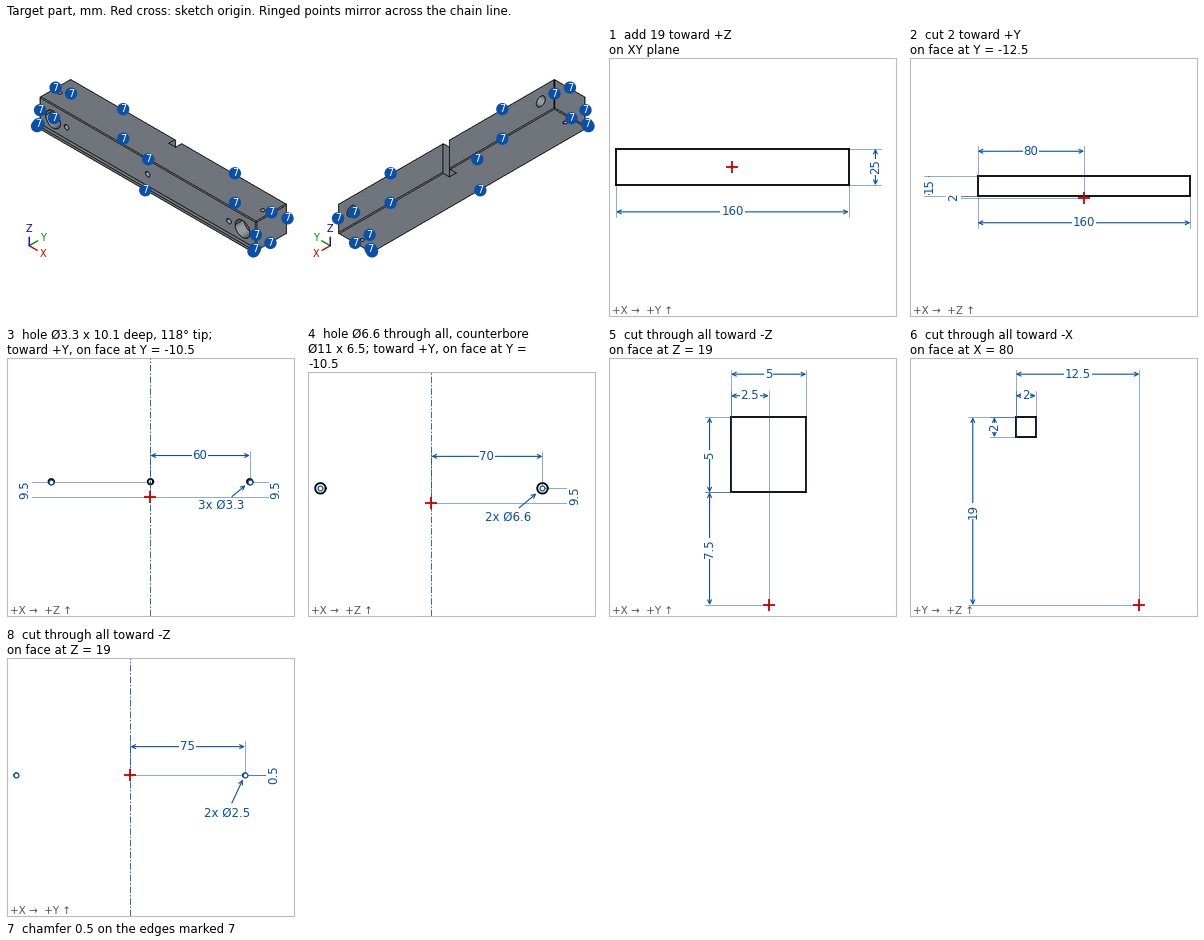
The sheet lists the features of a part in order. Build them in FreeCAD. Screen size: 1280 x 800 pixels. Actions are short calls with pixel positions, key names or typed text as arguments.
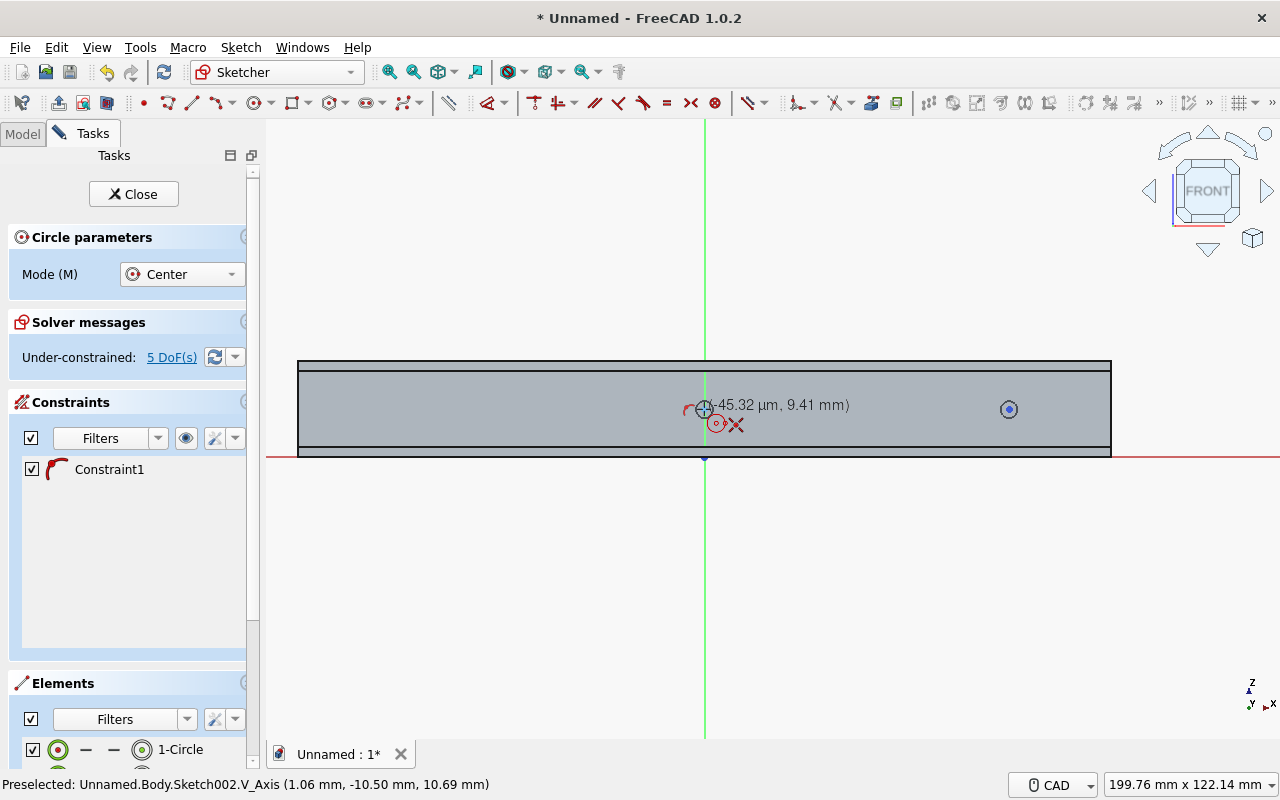
scroll(400, 409, up, 5)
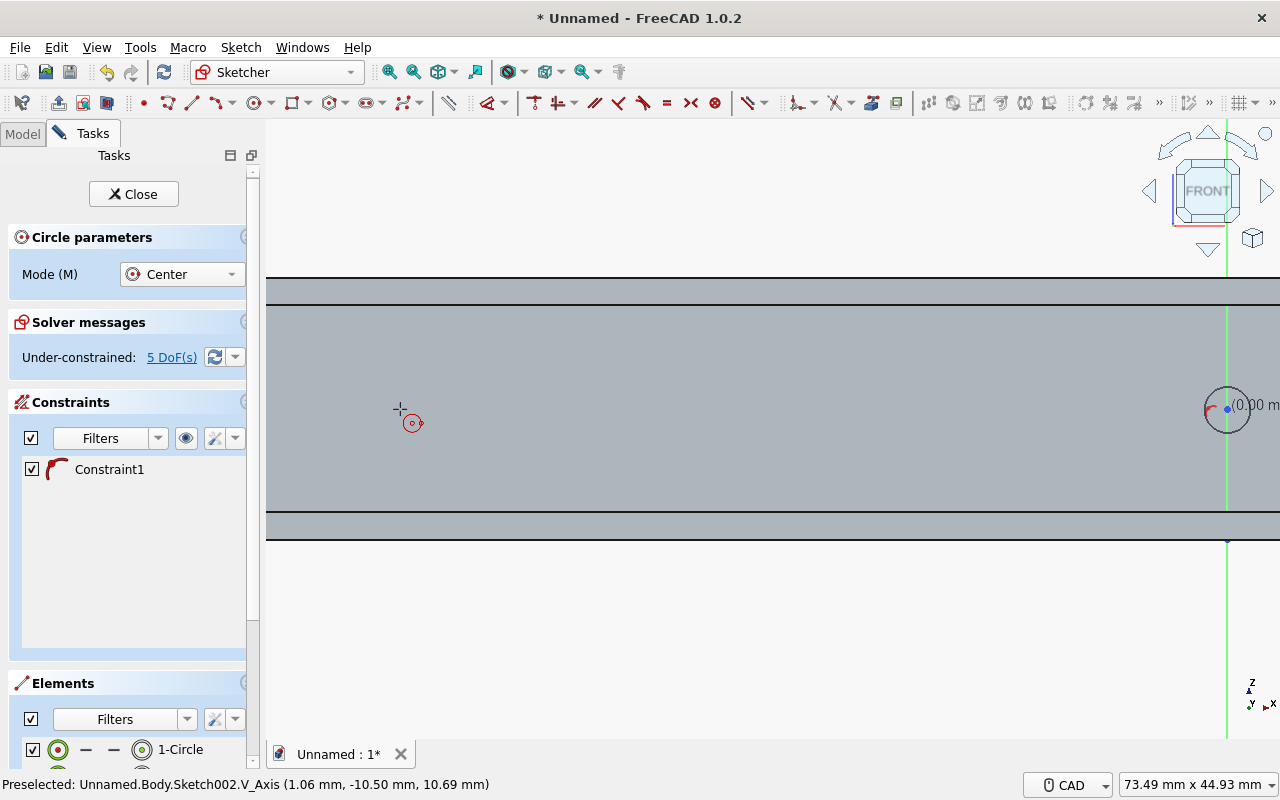
click(400, 409)
click(416, 393)
key(Escape)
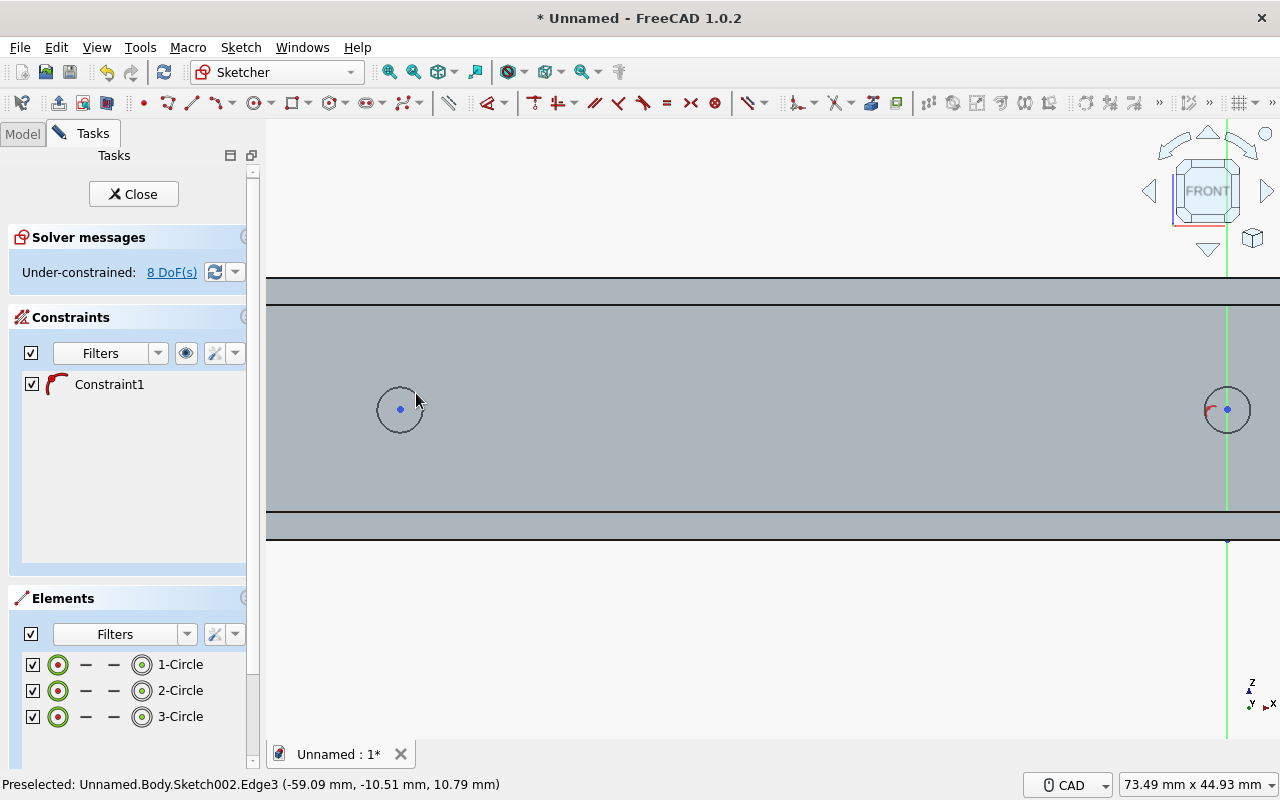
scroll(400, 409, down, 5)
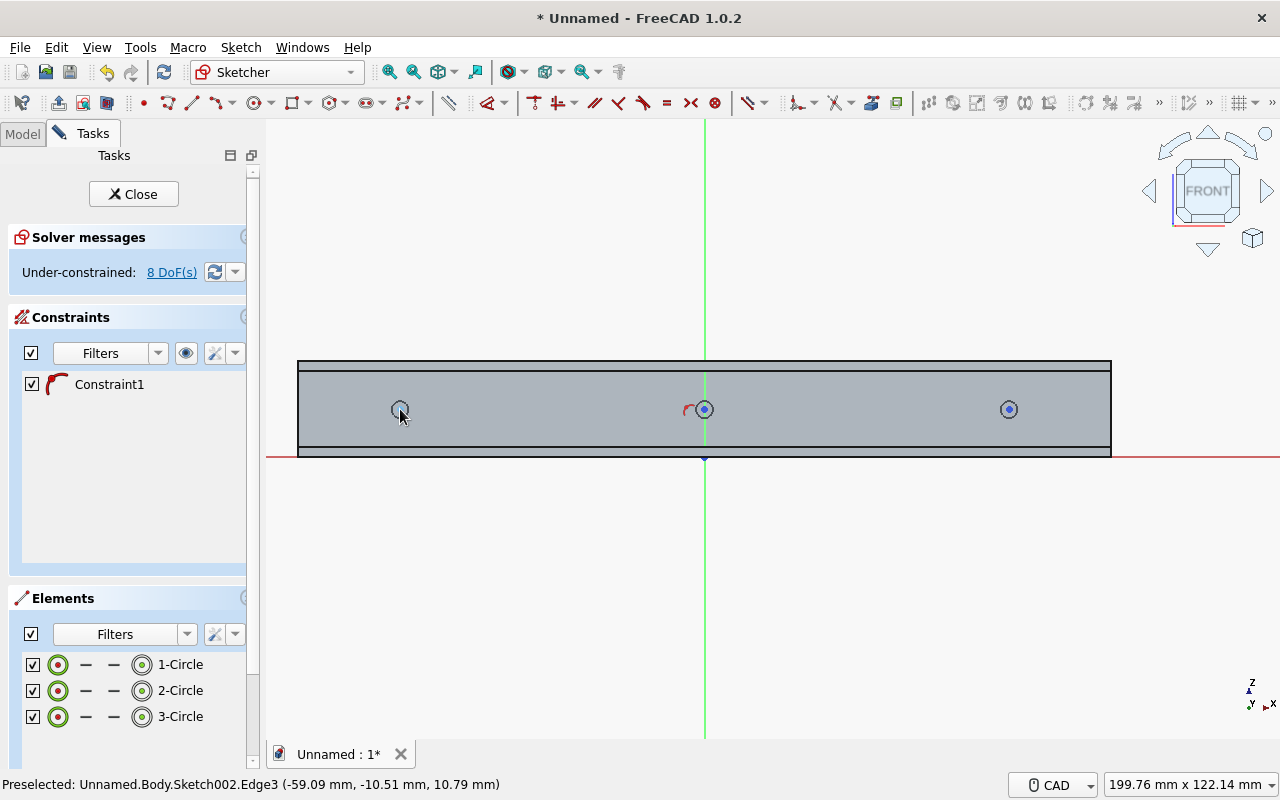
scroll(1015, 404, up, 3)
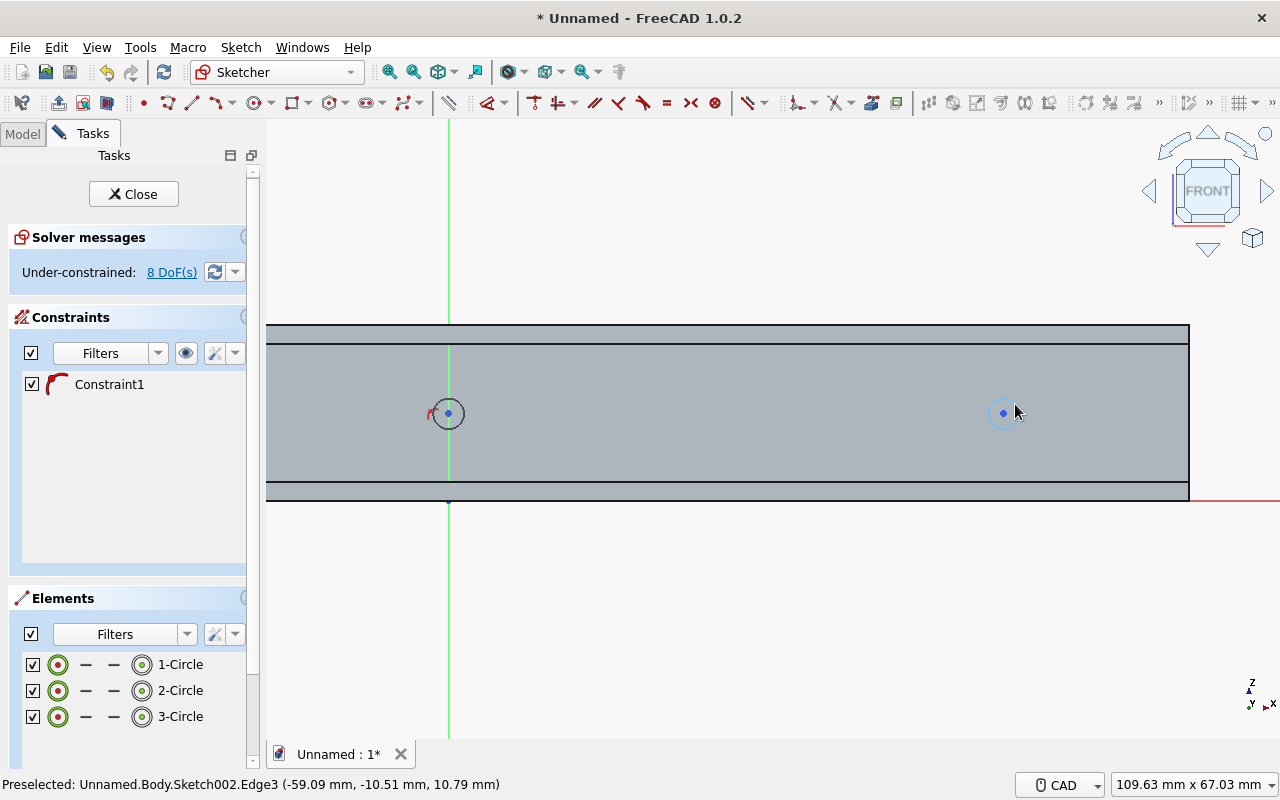
click(1014, 403)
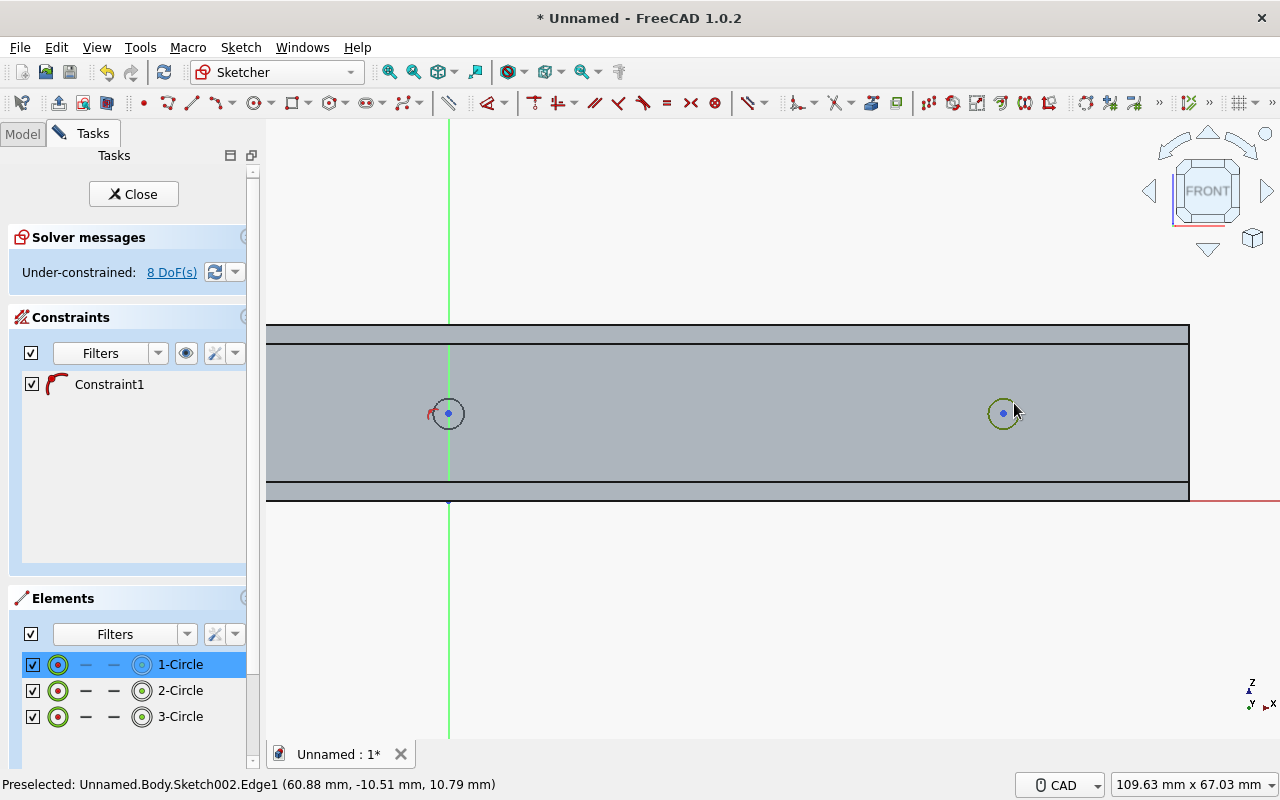
scroll(459, 403, up, 2)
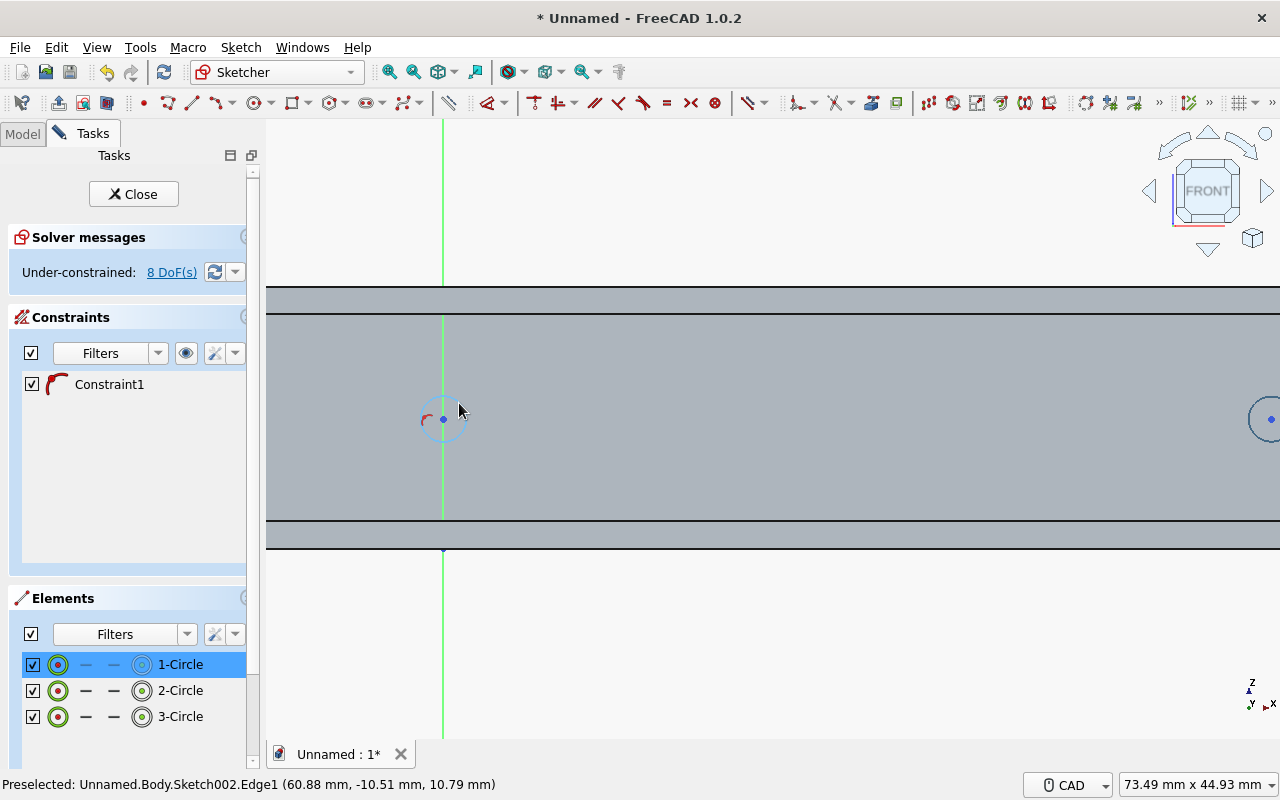
click(460, 403)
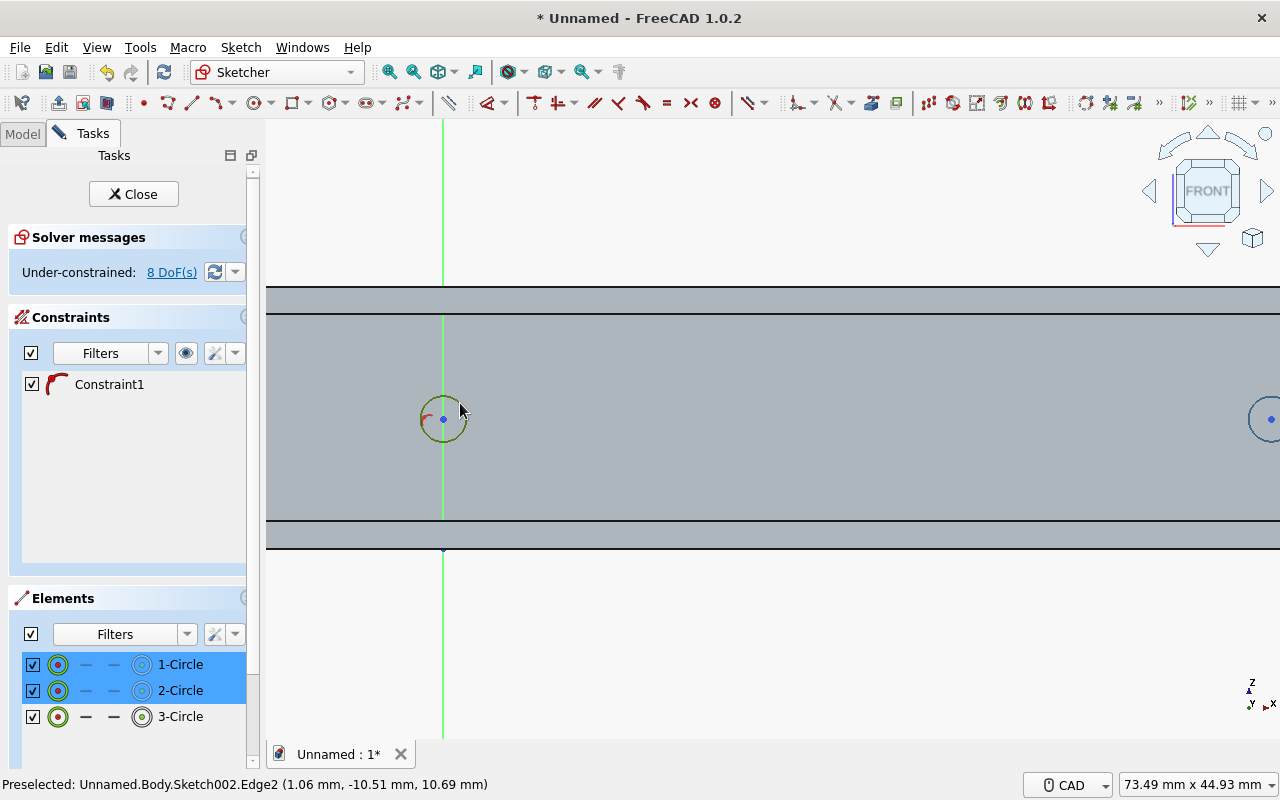
scroll(856, 404, down, 5)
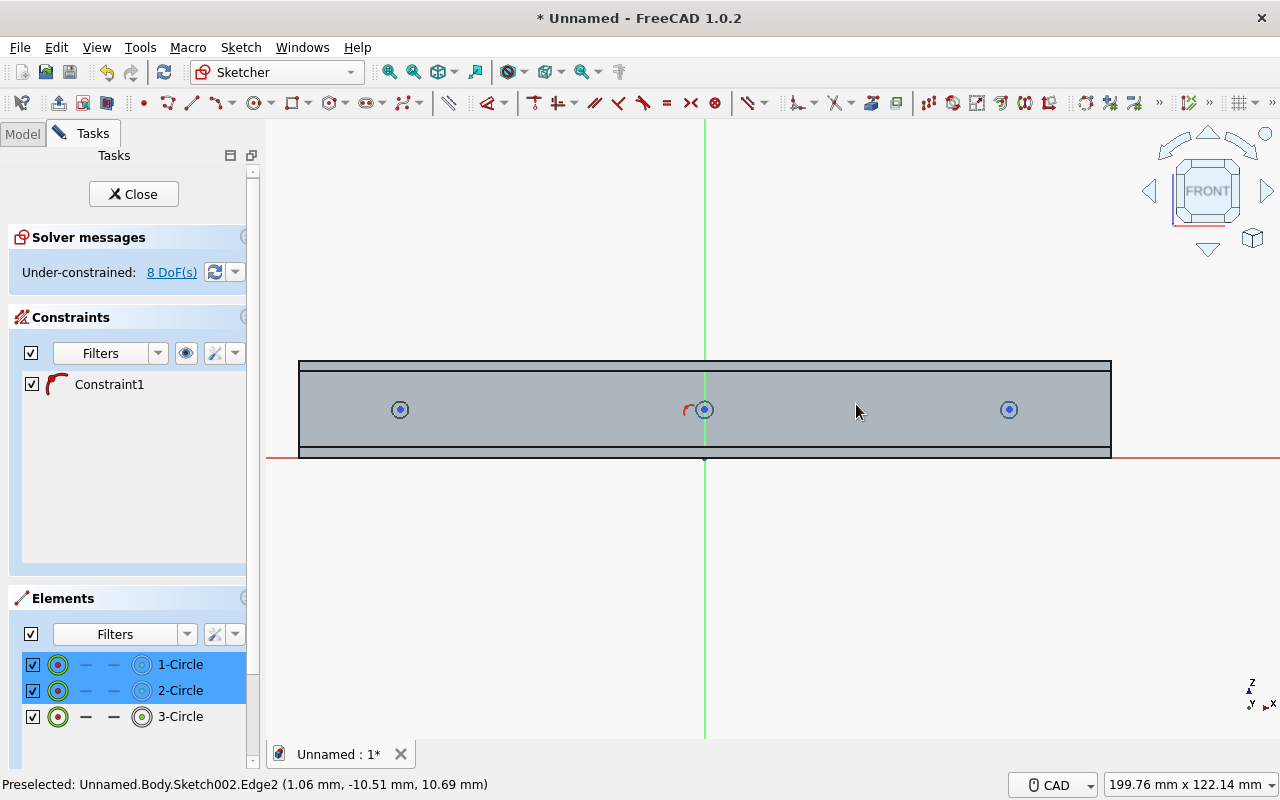
scroll(406, 404, up, 3)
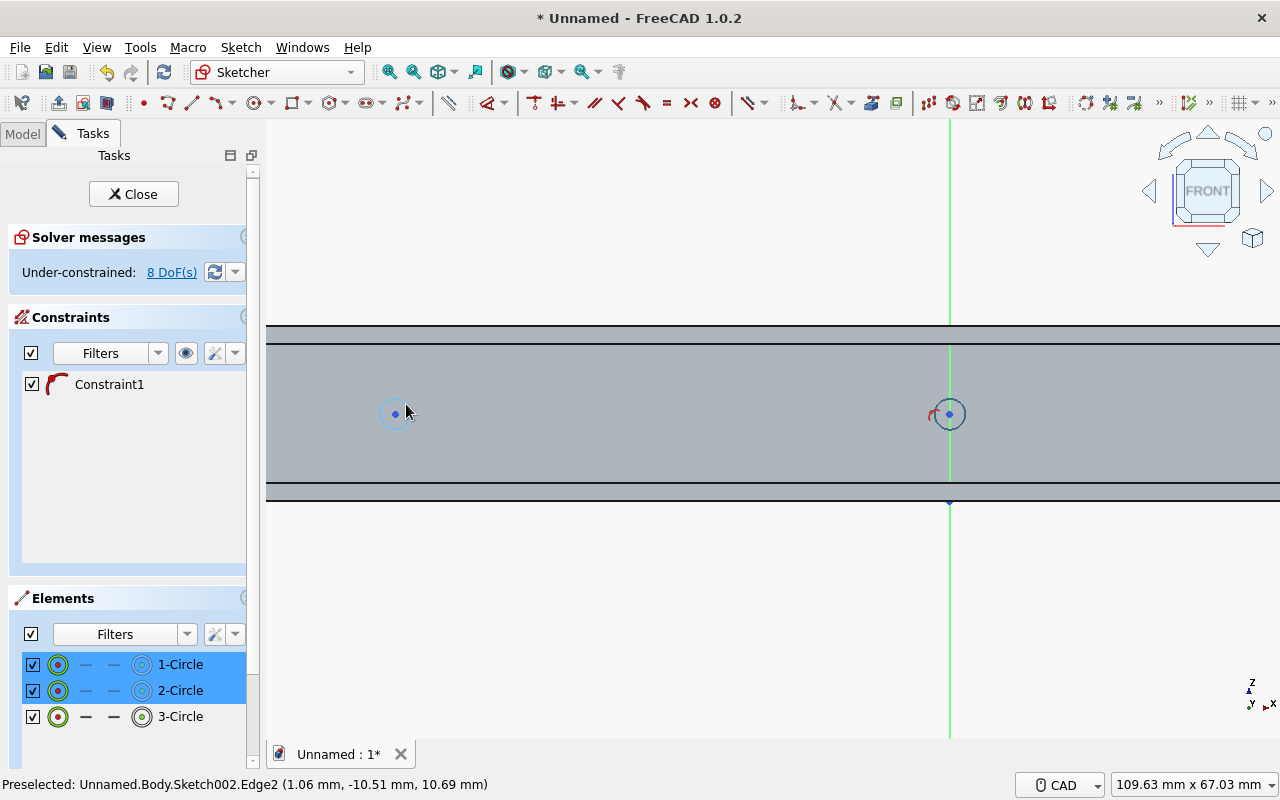
click(406, 404)